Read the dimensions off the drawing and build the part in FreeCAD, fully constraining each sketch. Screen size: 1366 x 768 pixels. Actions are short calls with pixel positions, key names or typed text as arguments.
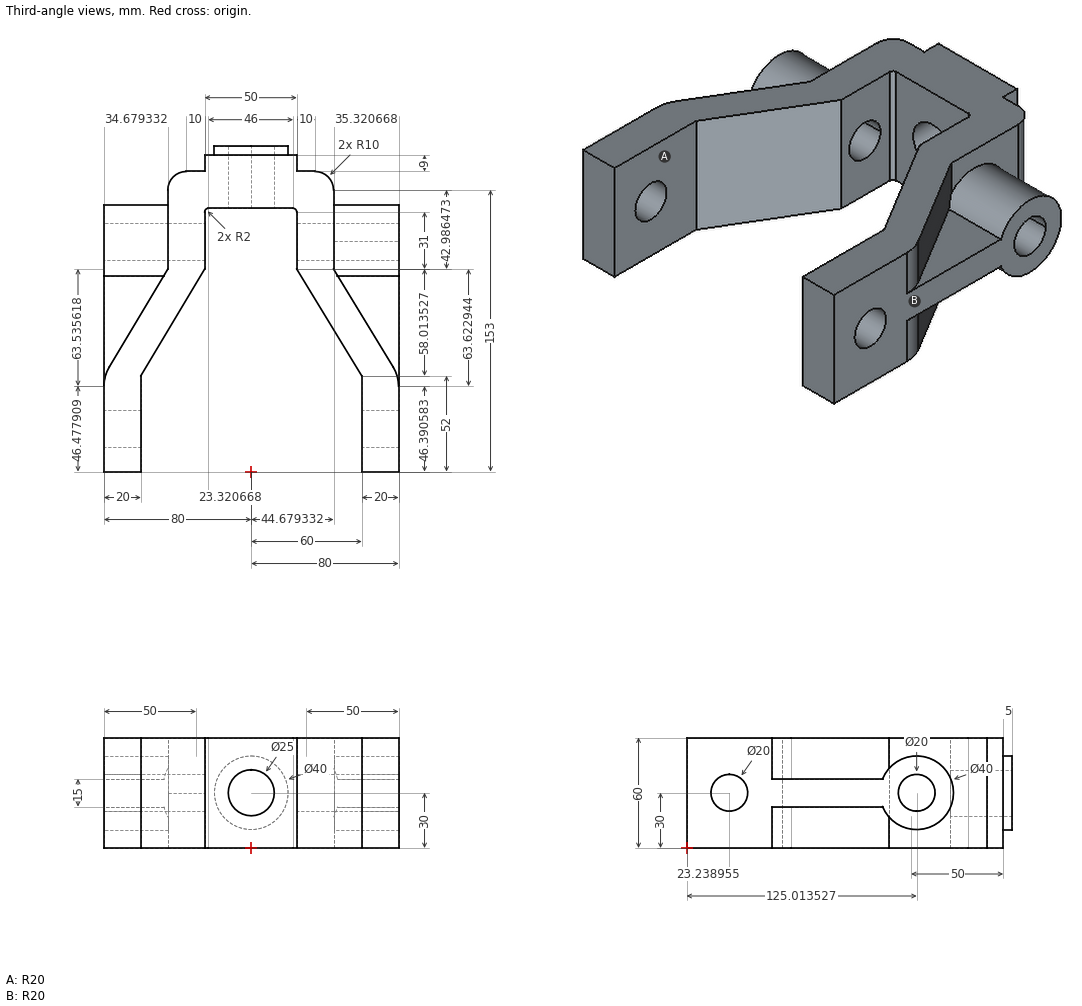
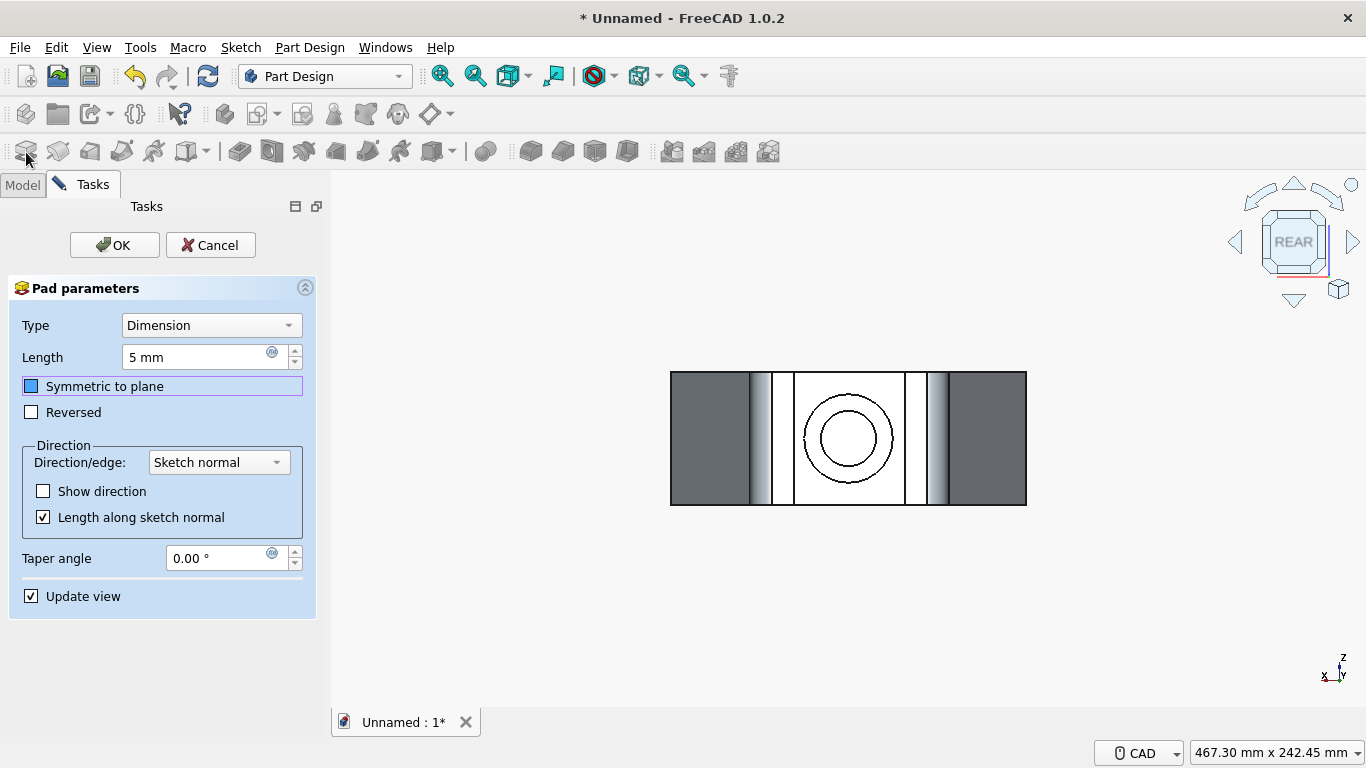
click(115, 245)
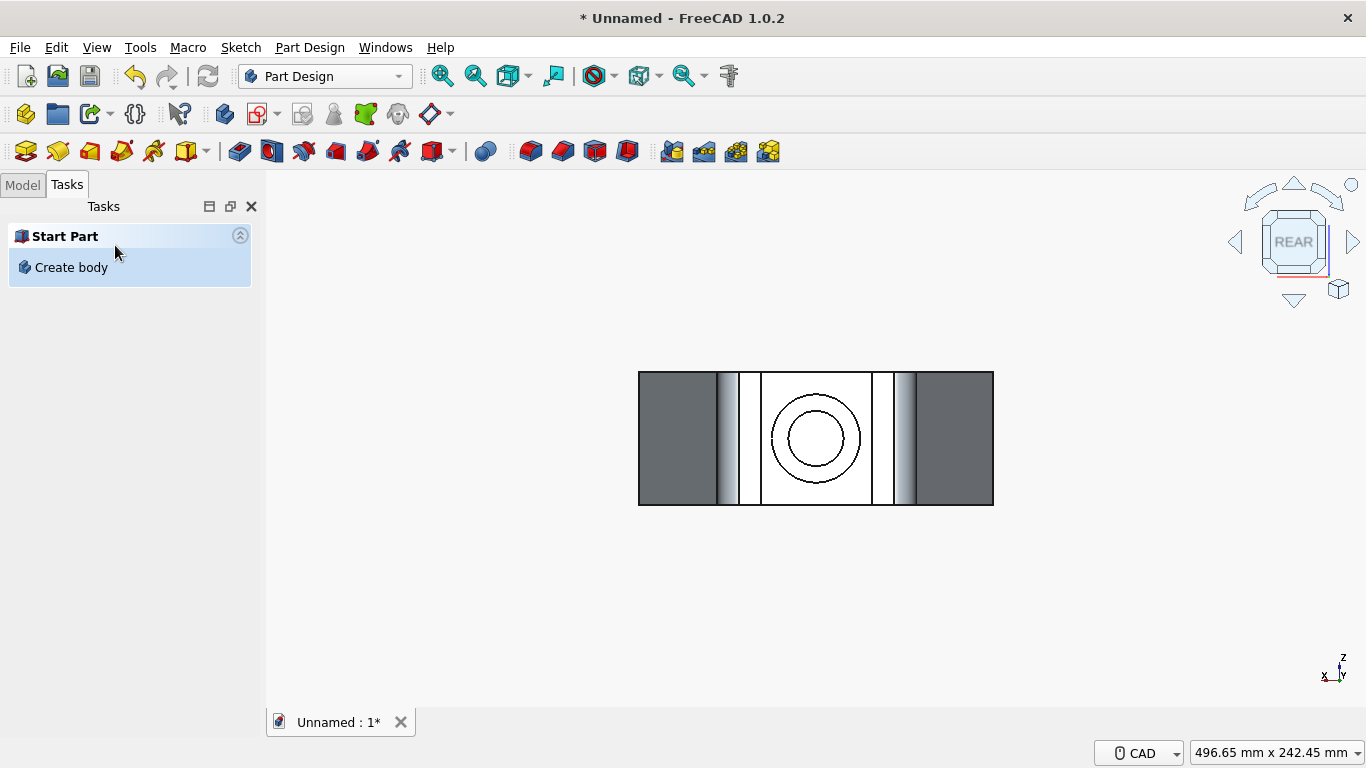
click(444, 76)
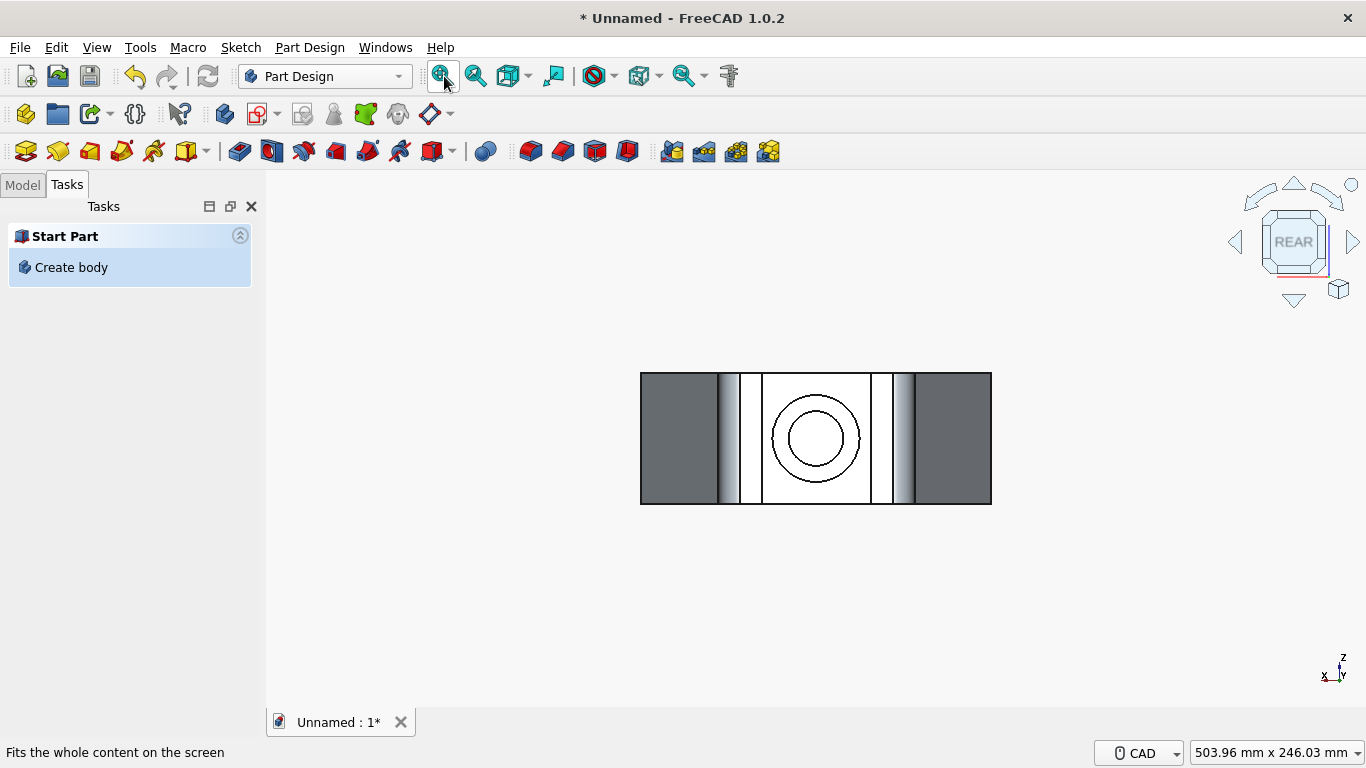
click(23, 184)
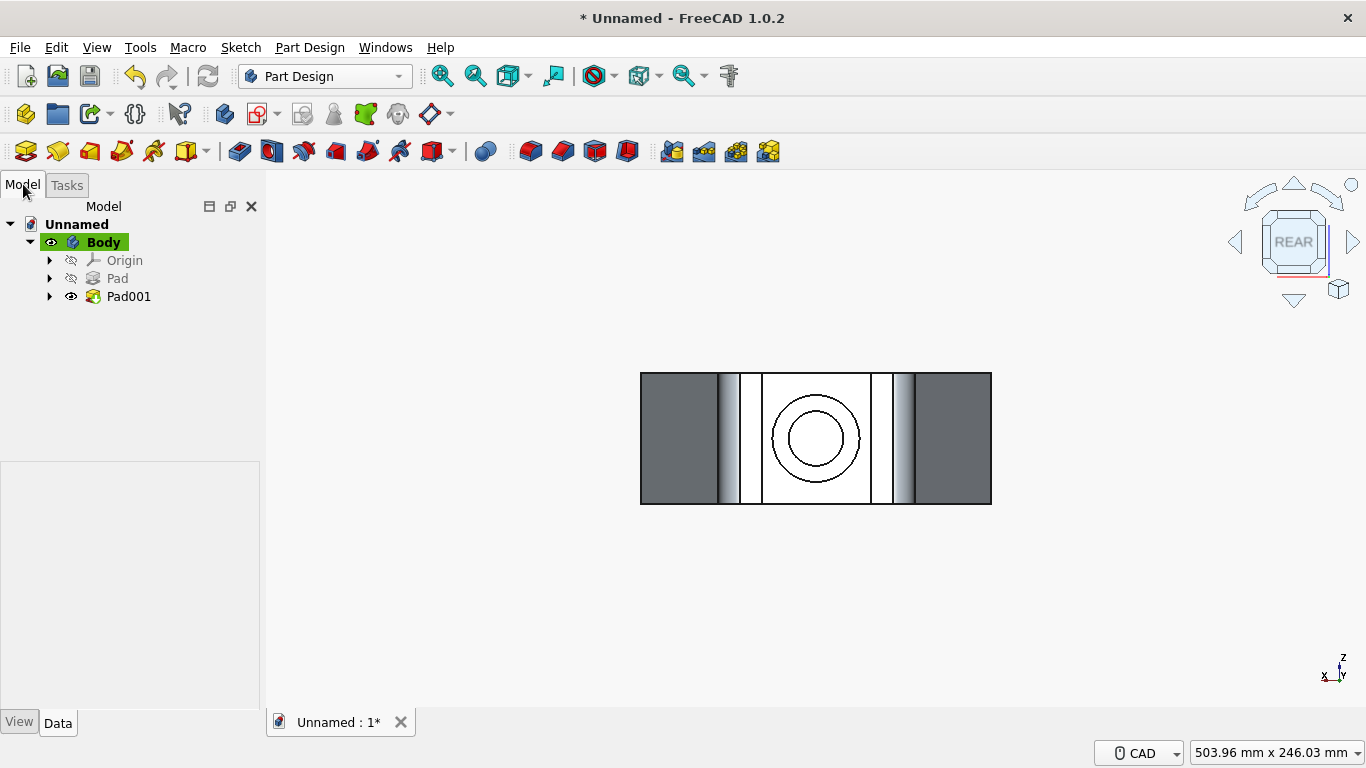
click(50, 260)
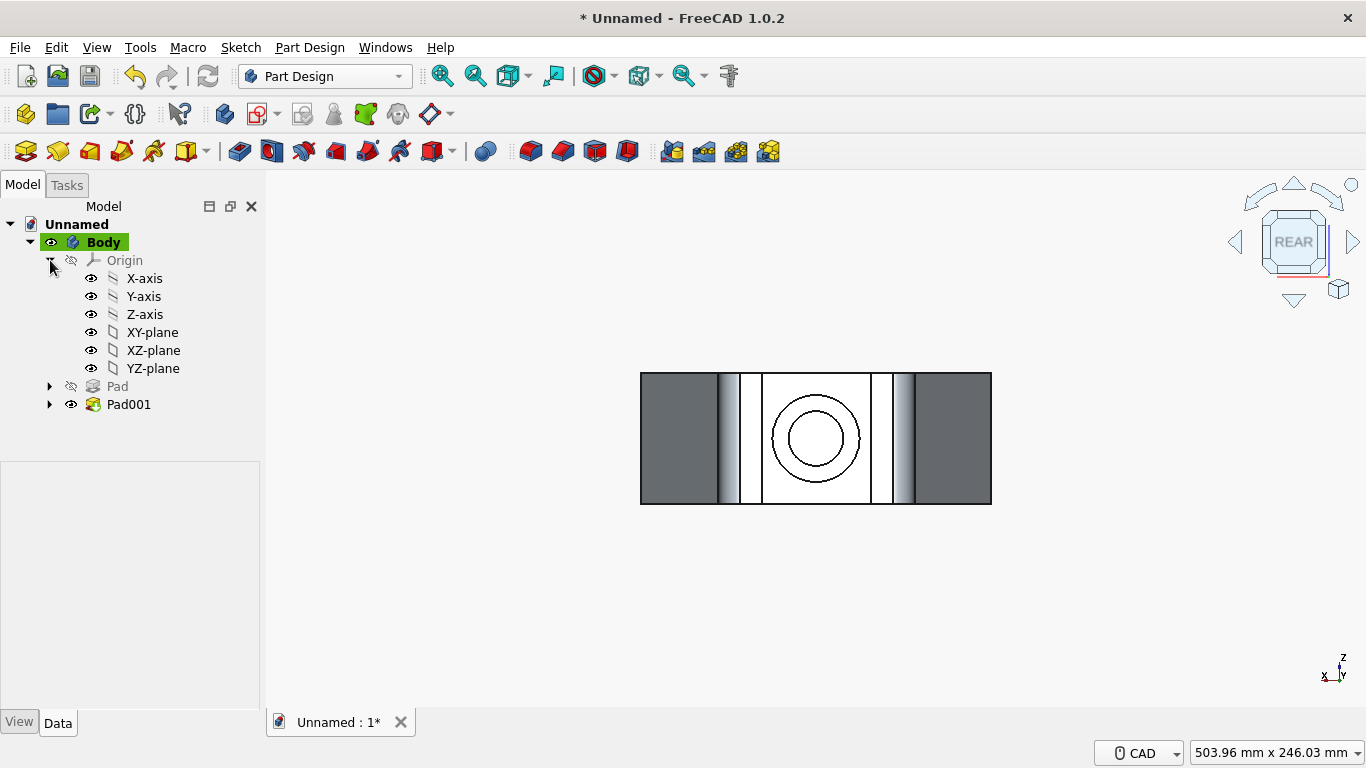
click(136, 350)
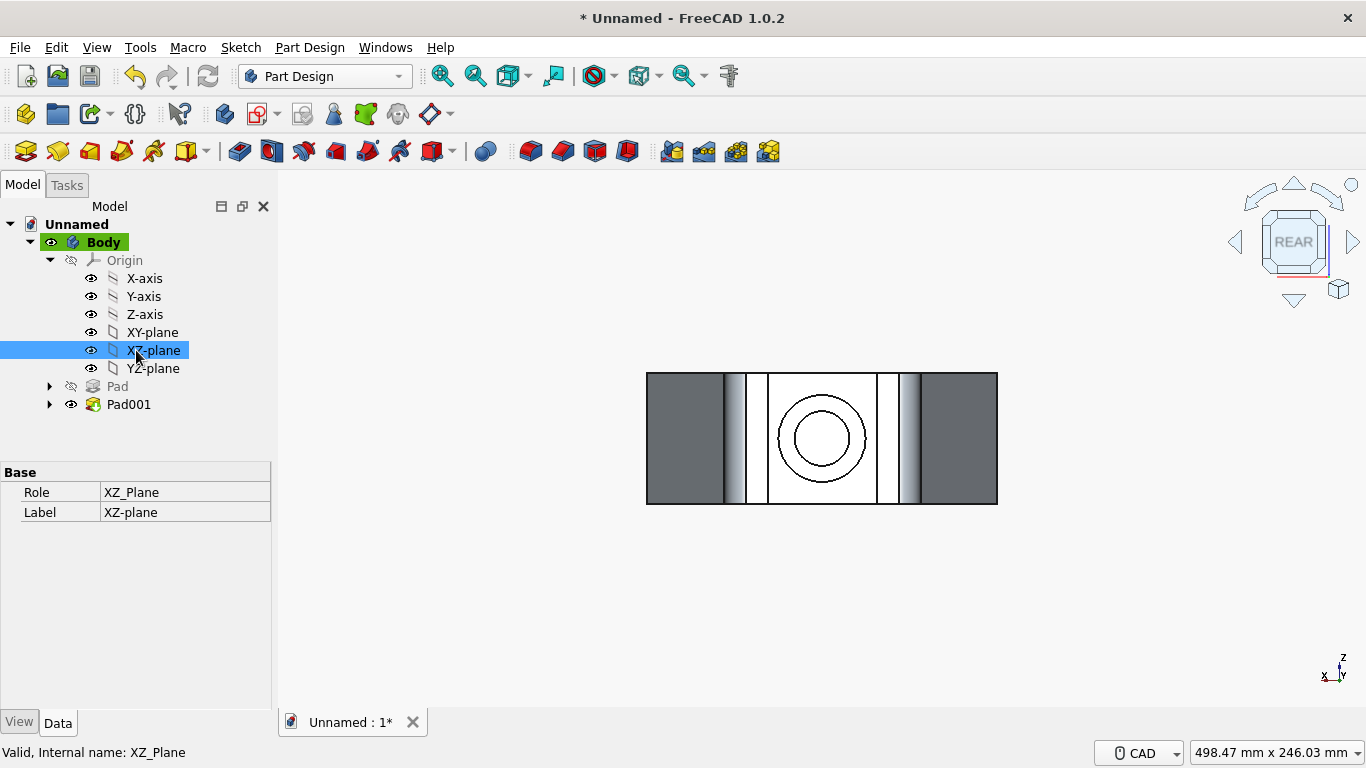
click(430, 114)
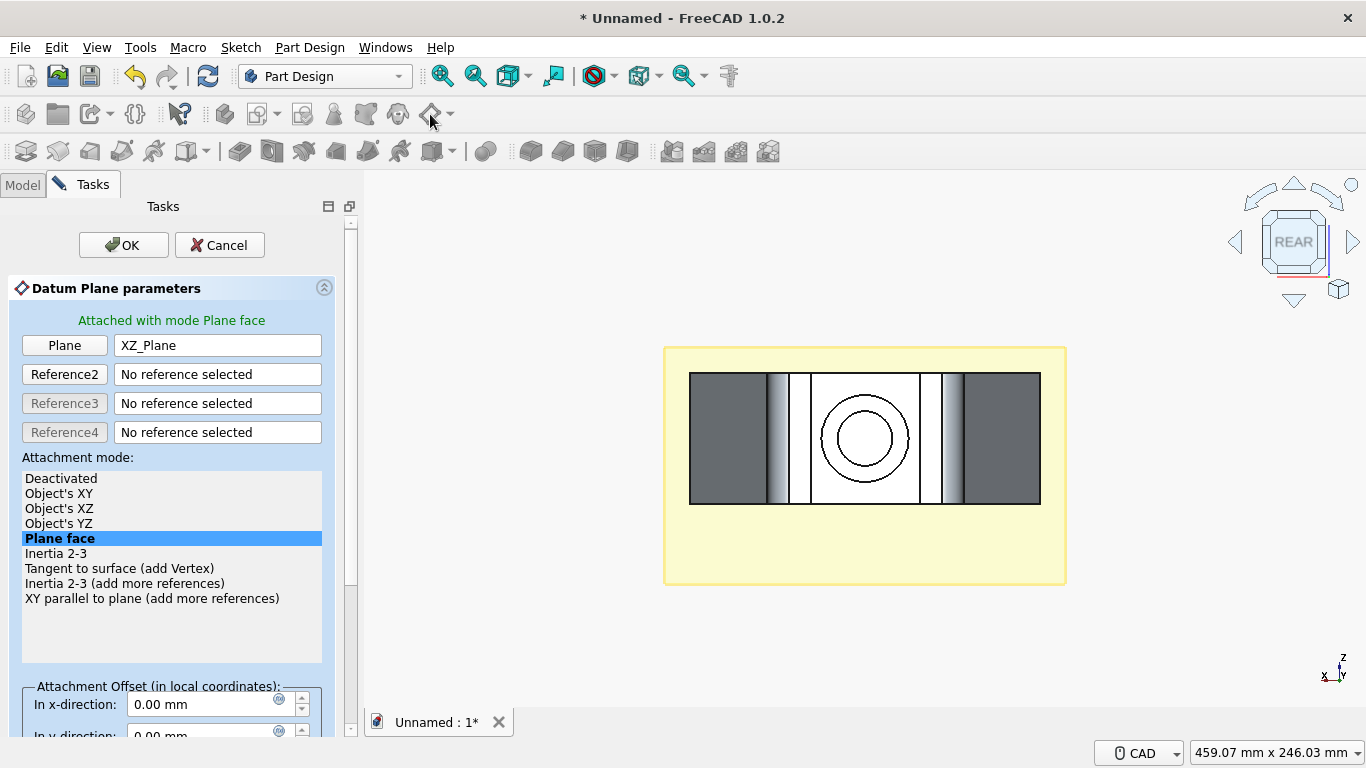
scroll(351, 476, down, 2)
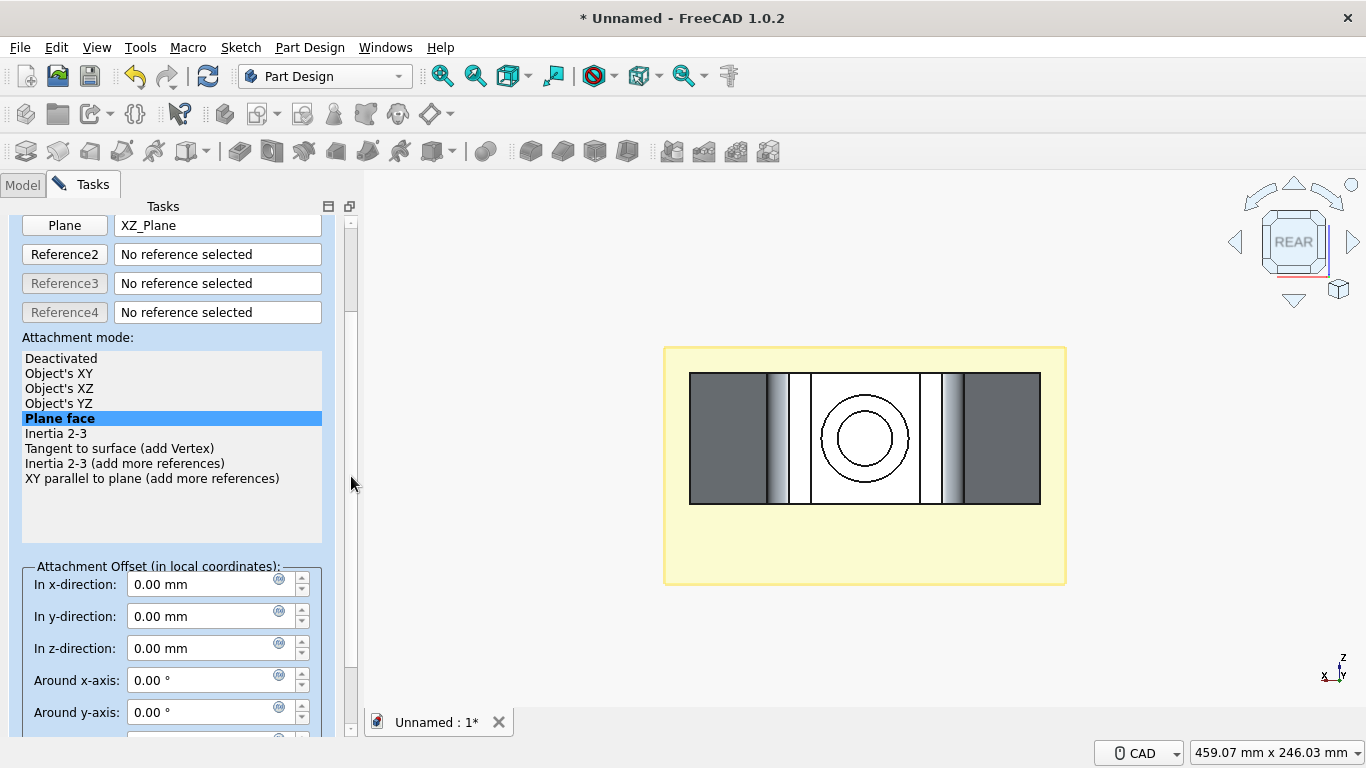
triple_click(210, 648)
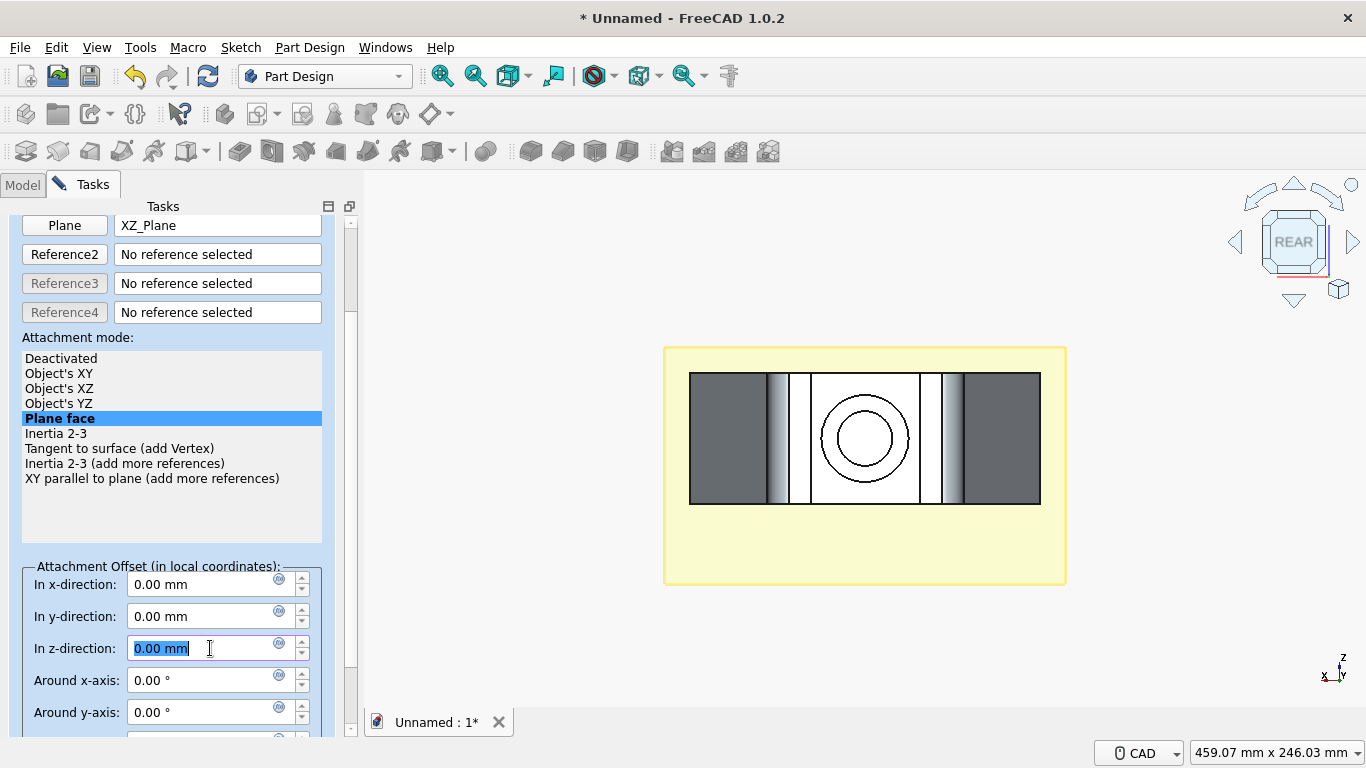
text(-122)
key(Tab)